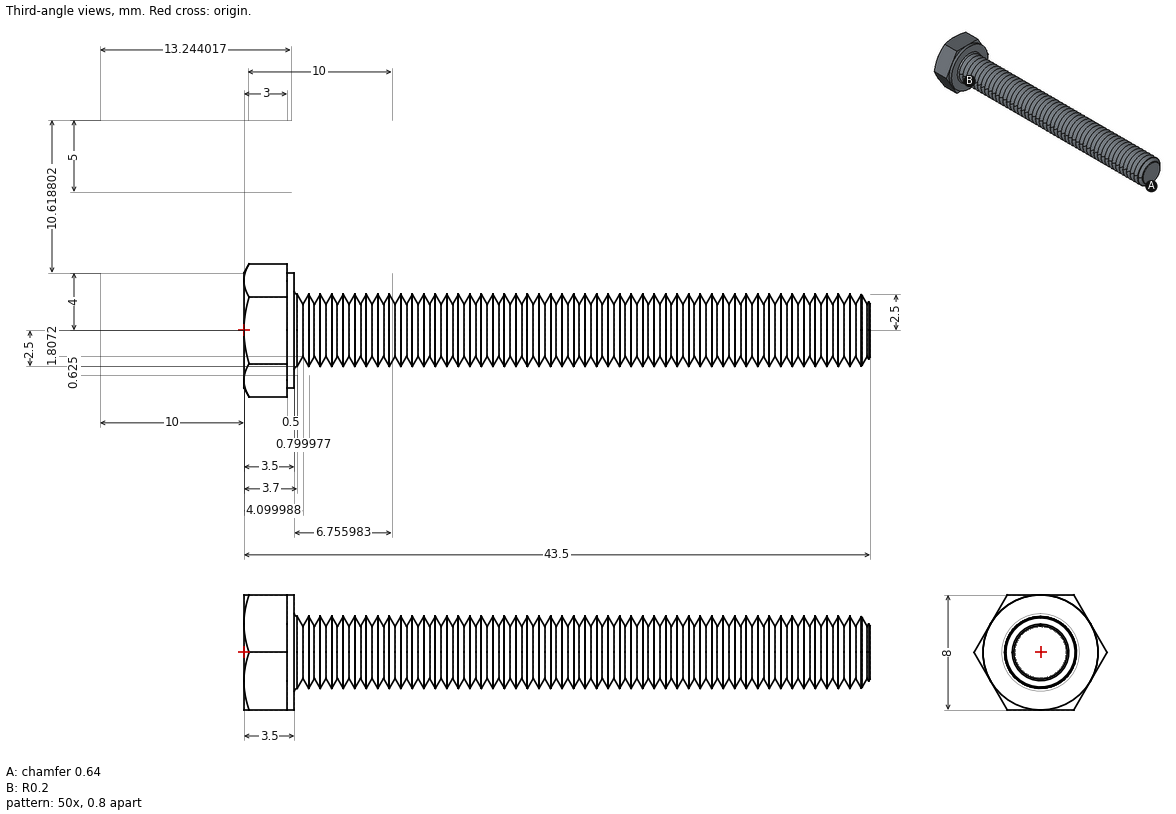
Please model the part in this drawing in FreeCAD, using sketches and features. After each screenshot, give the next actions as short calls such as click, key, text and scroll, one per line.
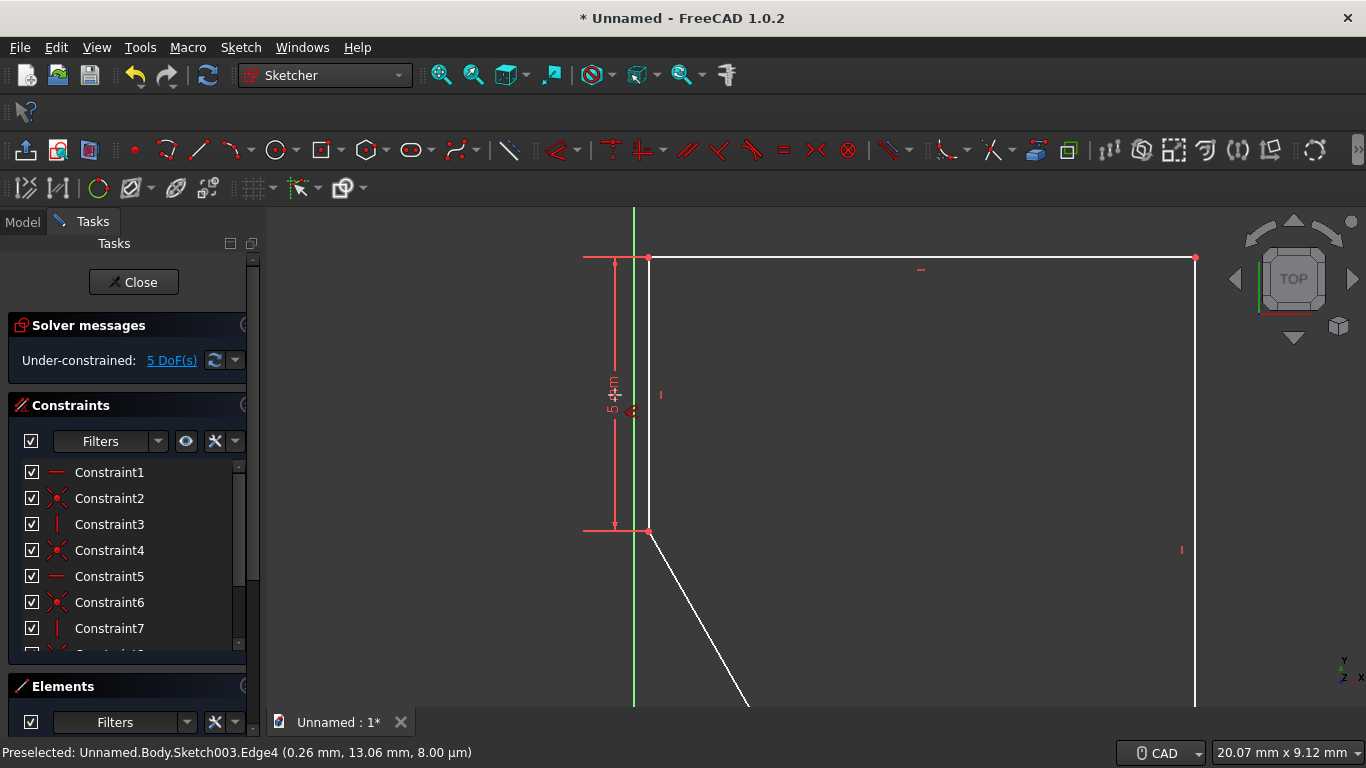
click(1031, 257)
click(922, 291)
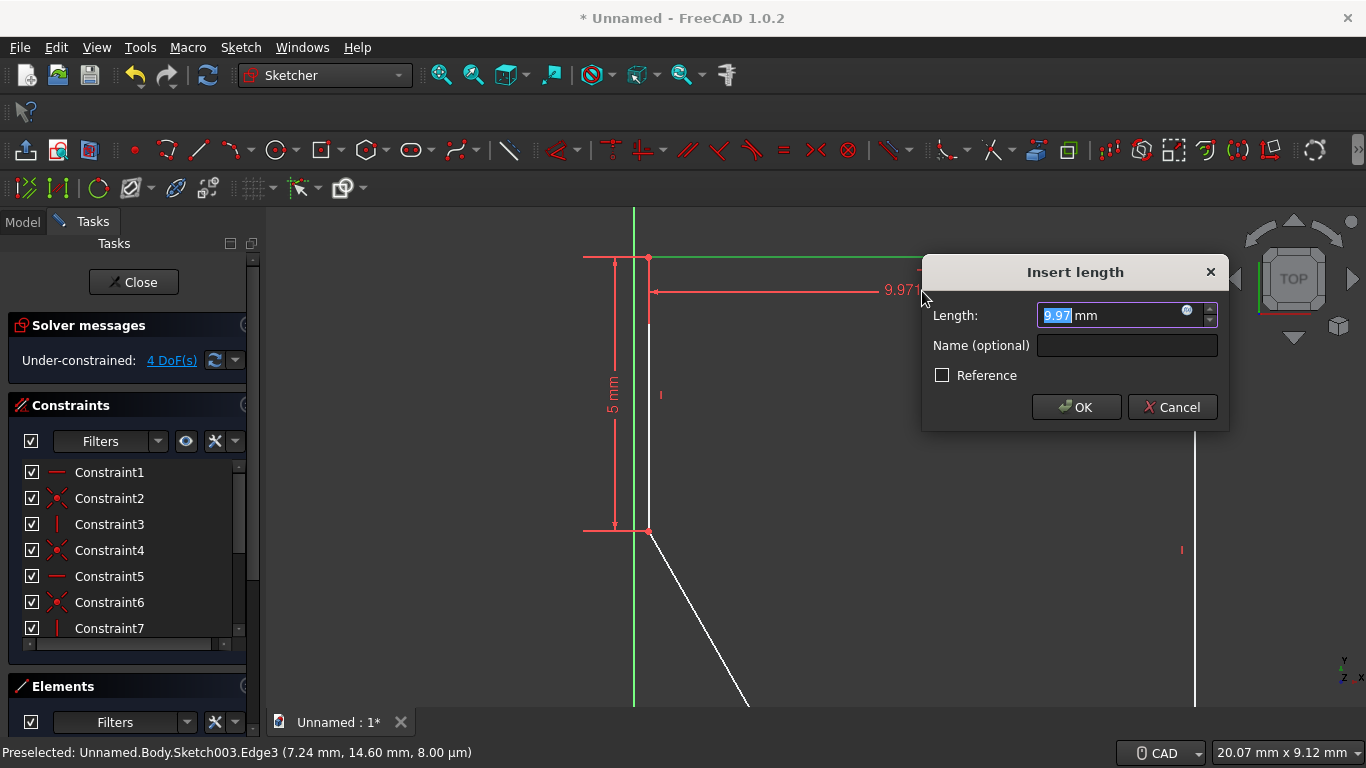
text(10)
key(Return)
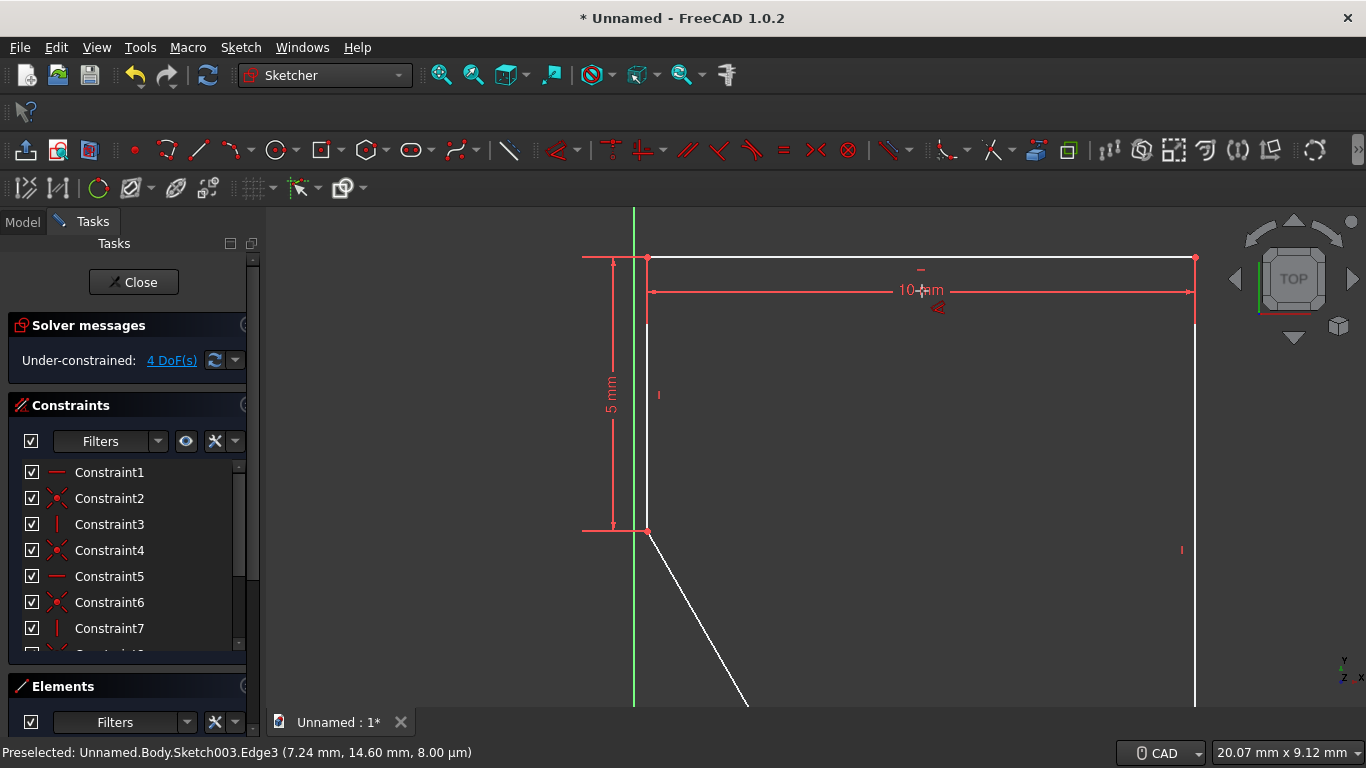
scroll(650, 341, down, 5)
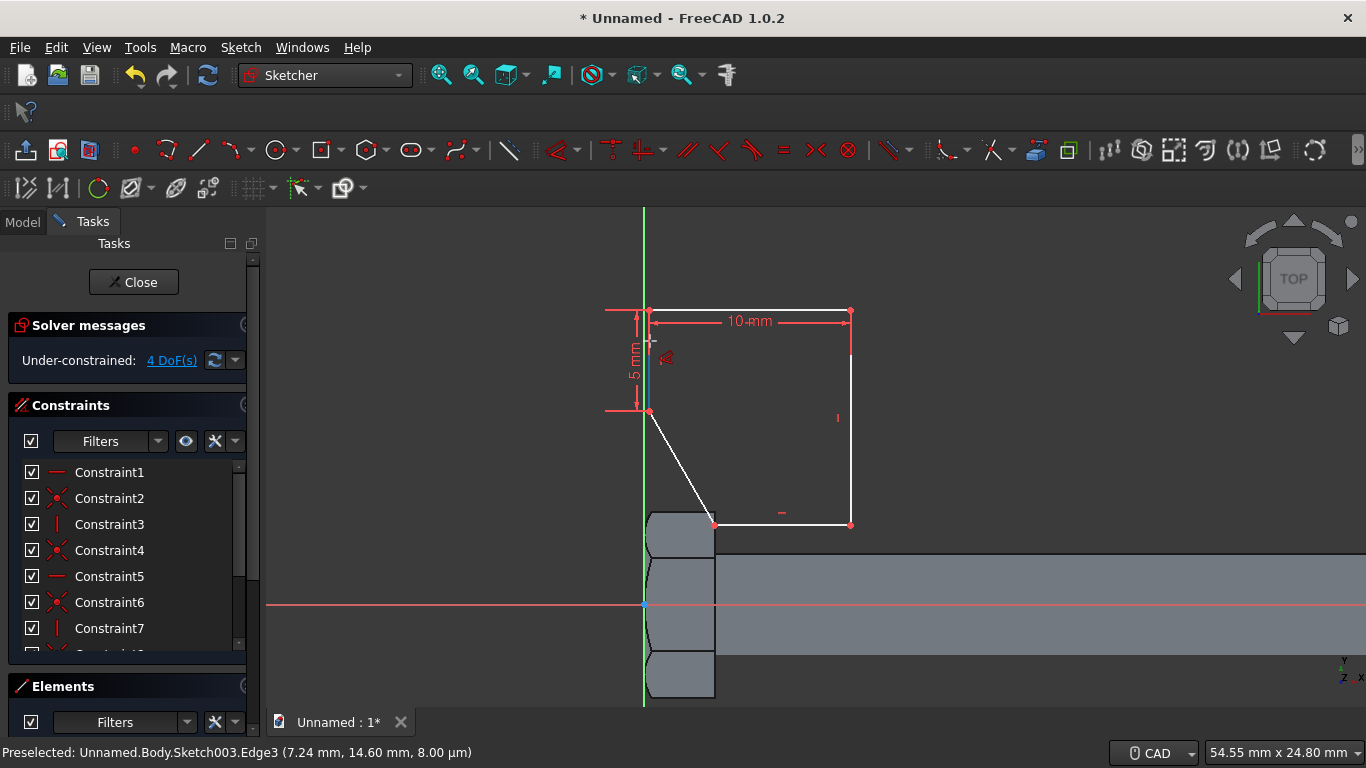
click(715, 525)
click(610, 565)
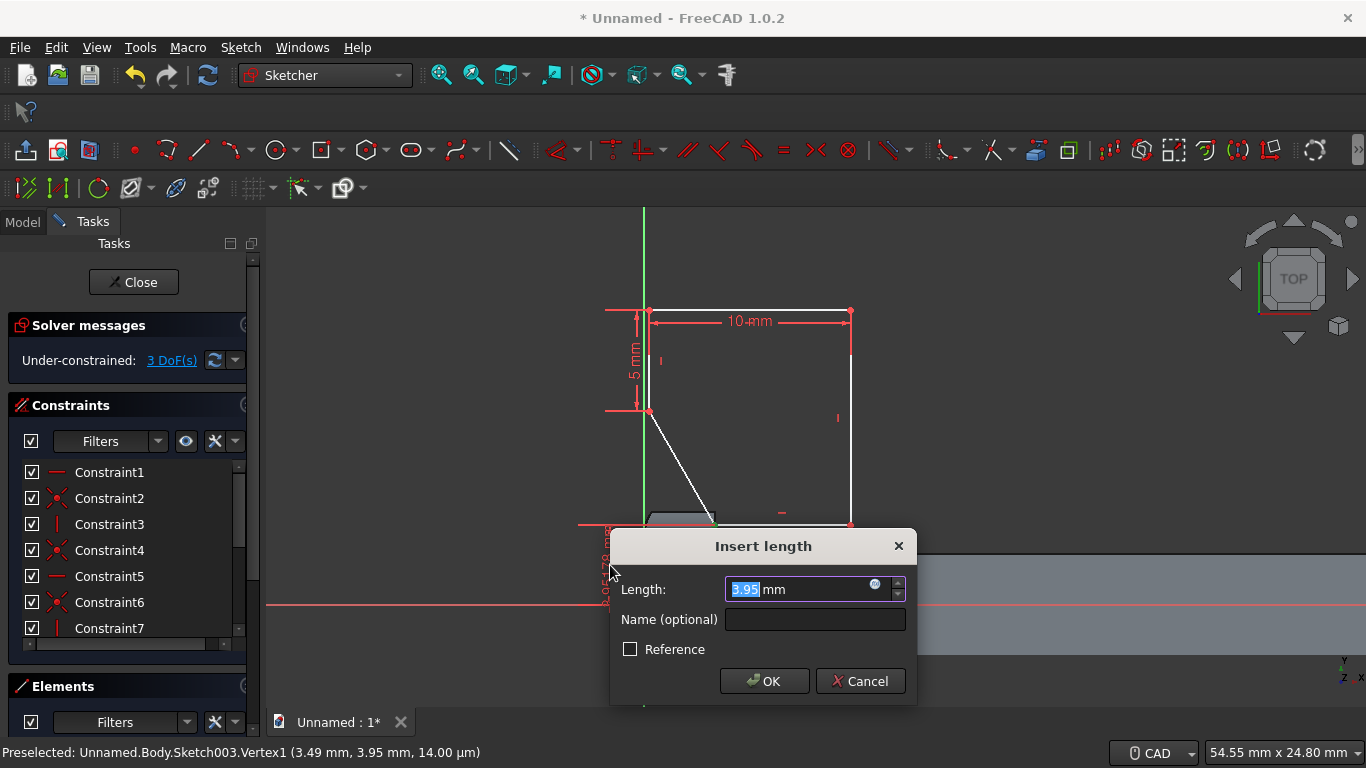
text(4)
key(Return)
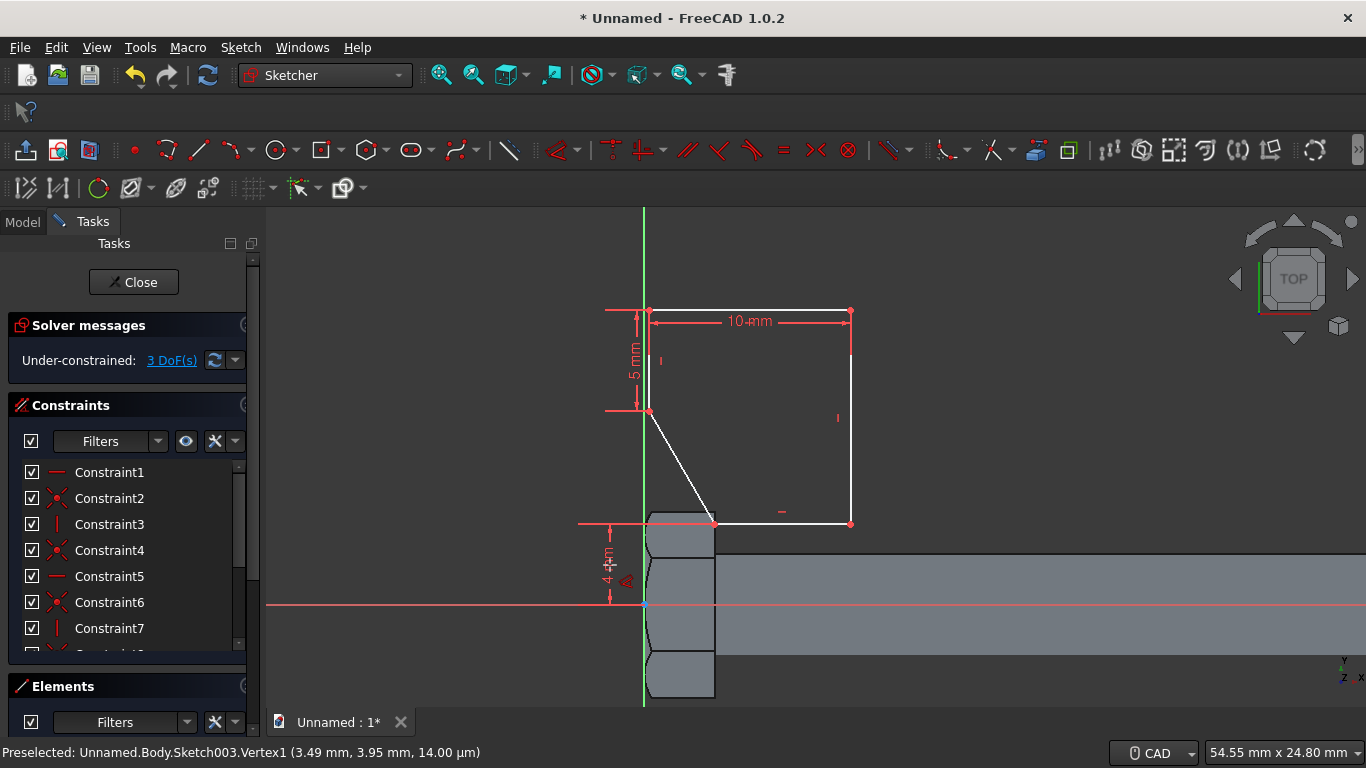
click(715, 524)
click(680, 639)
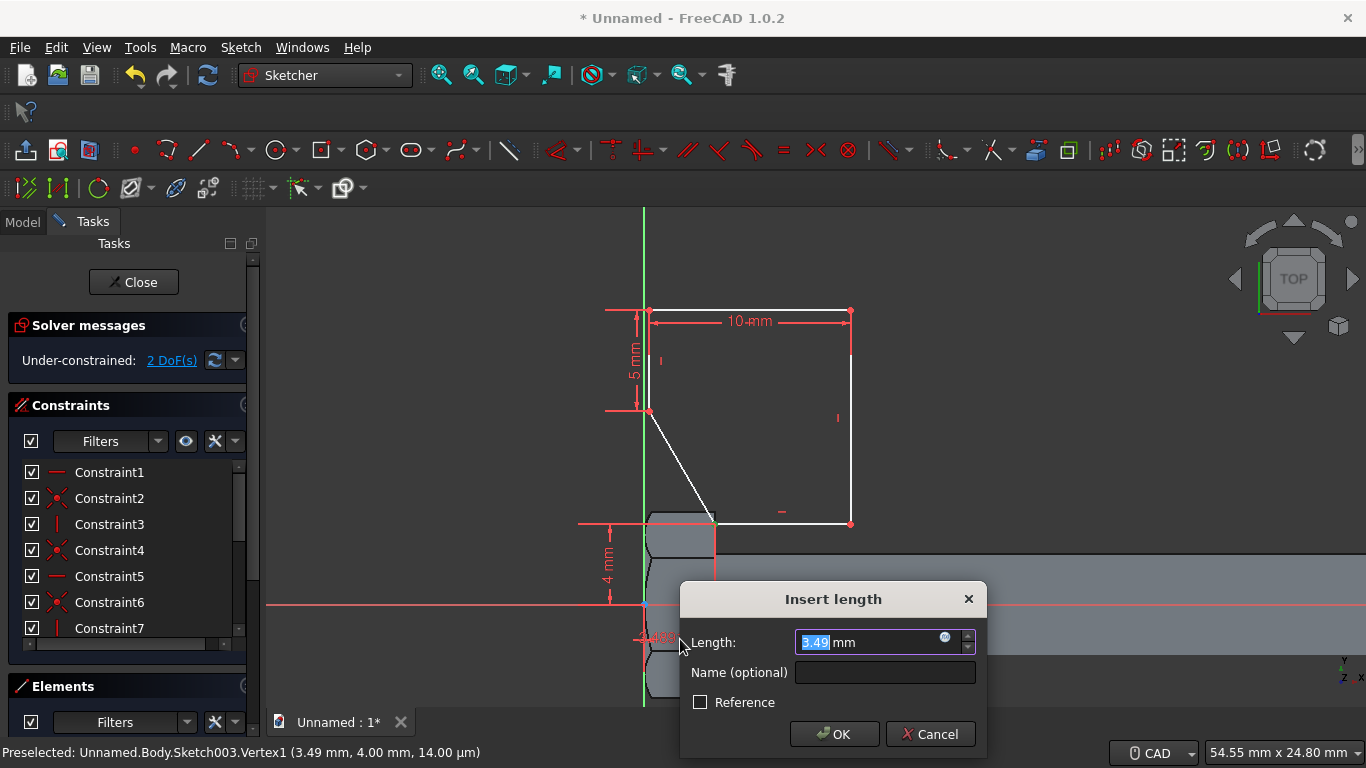
text(3.5)
key(Return)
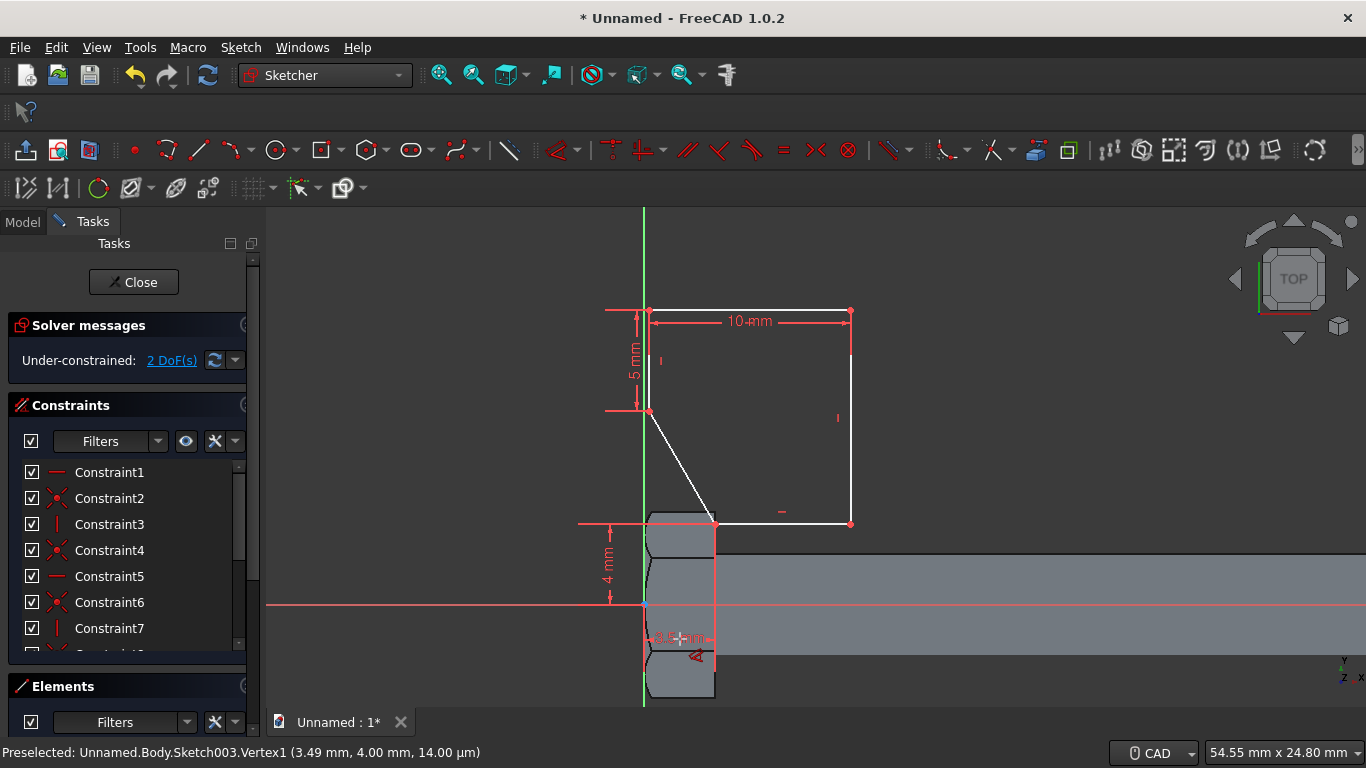
click(756, 524)
click(783, 558)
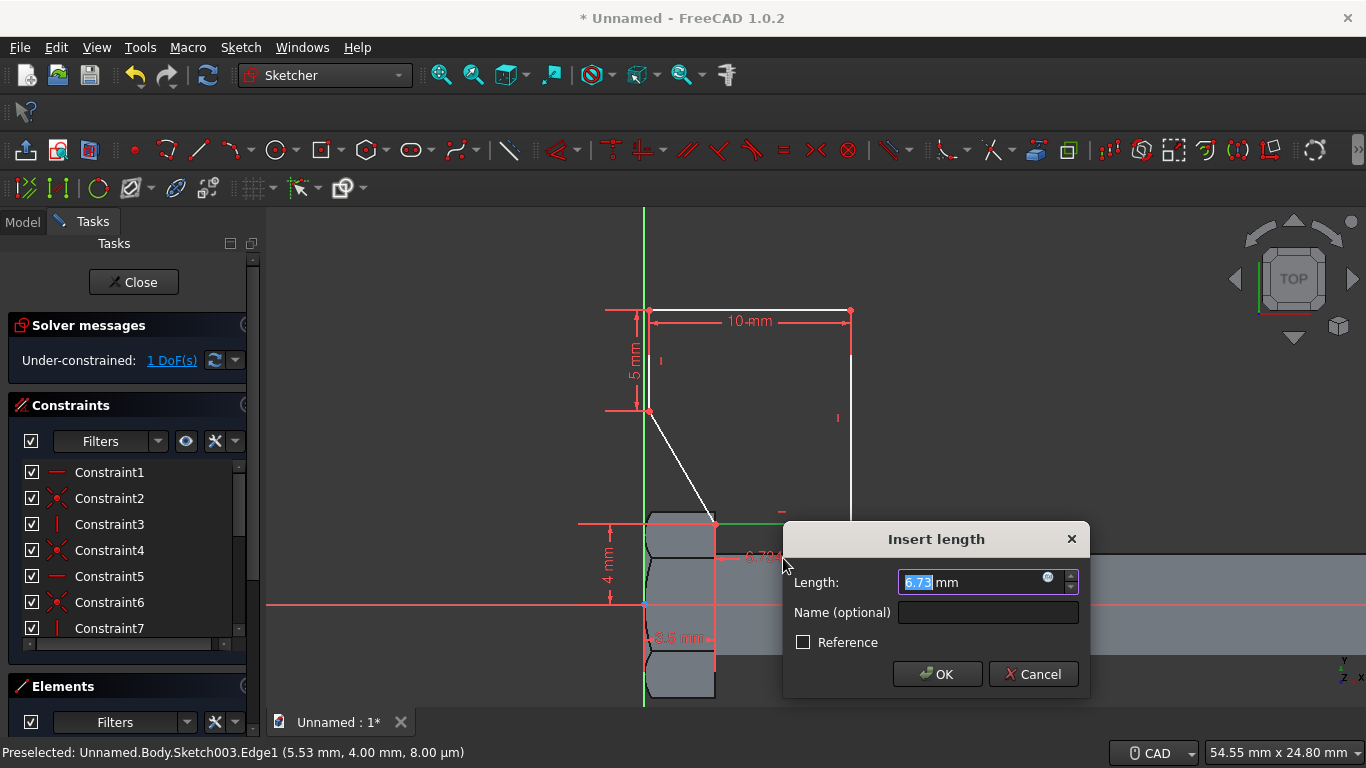
text(6.755983)
key(Return)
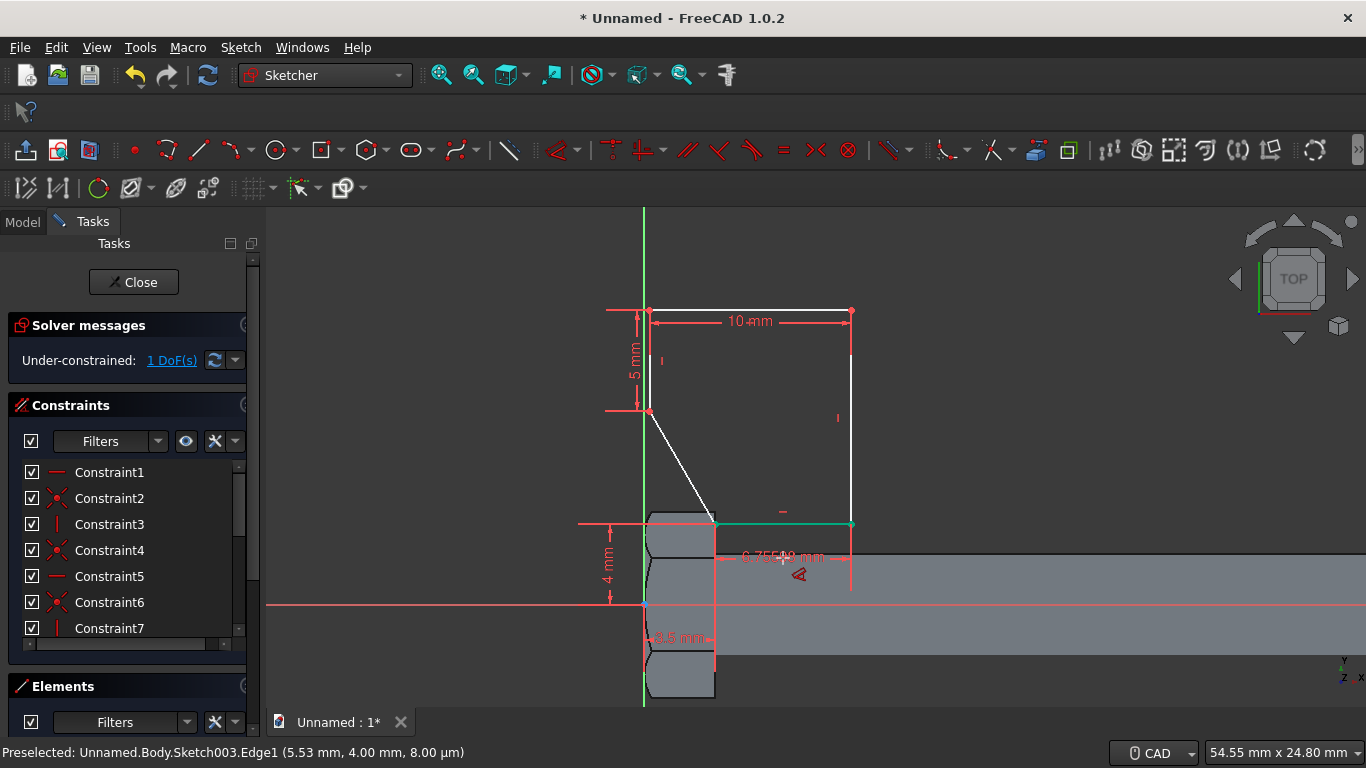
click(851, 460)
click(885, 417)